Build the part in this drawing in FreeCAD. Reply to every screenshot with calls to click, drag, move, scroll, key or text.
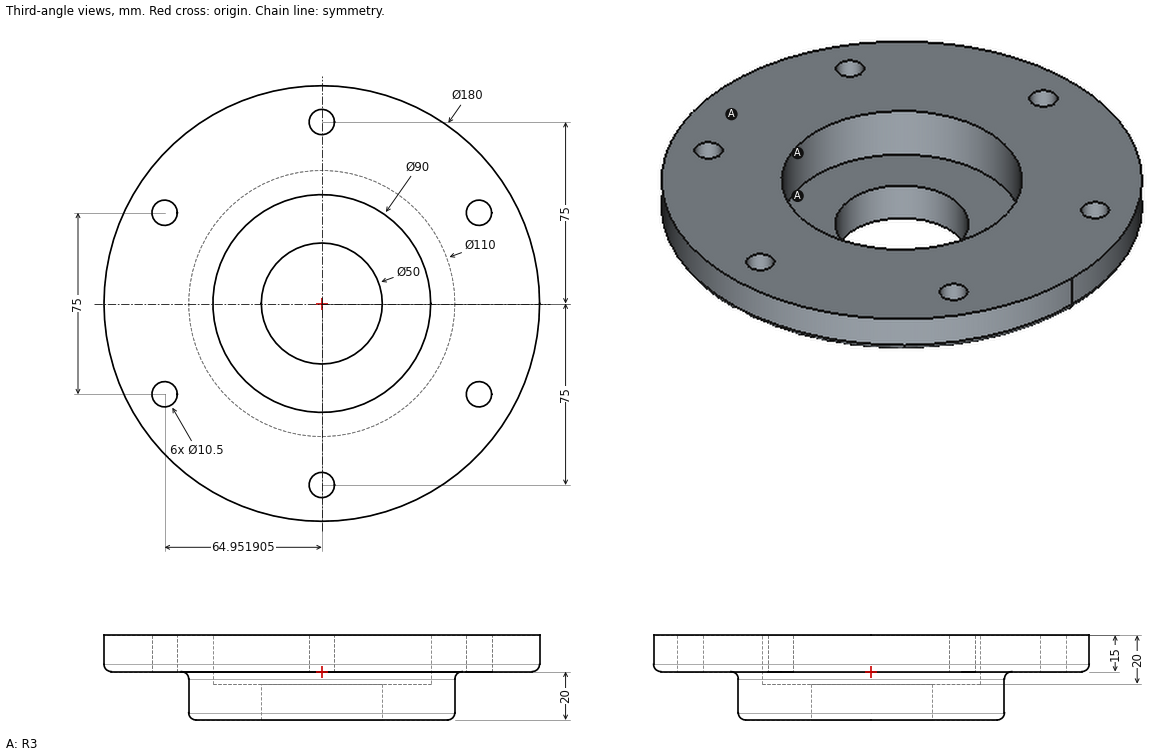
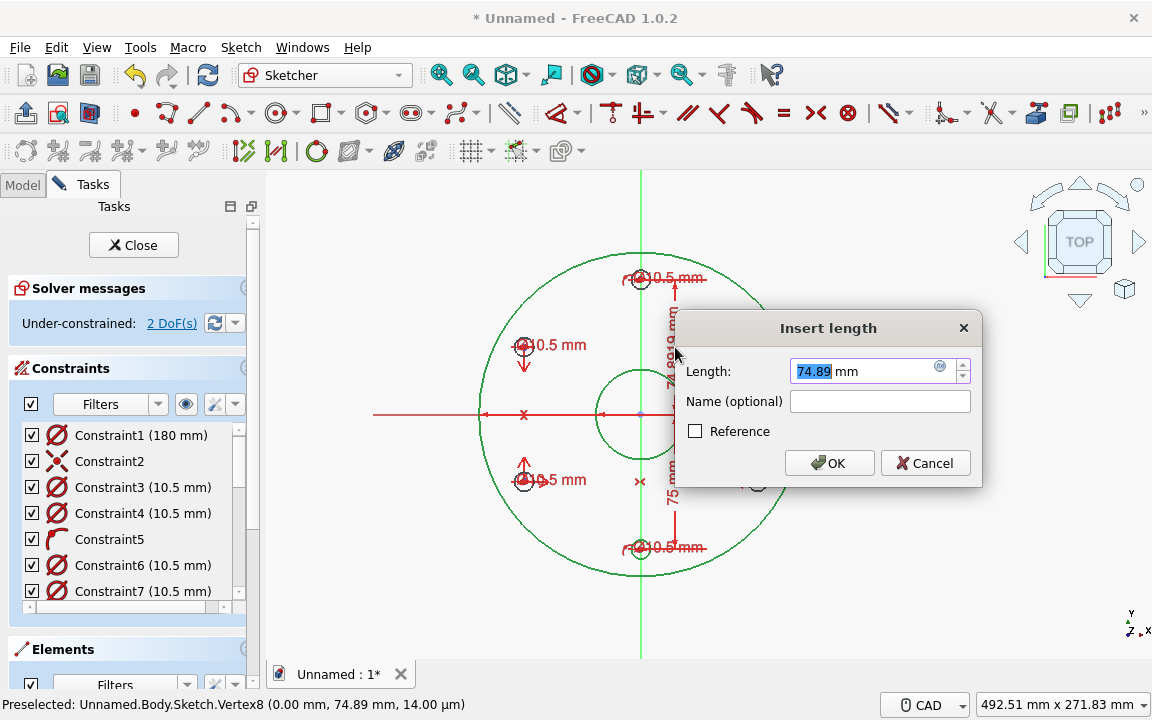
text(75)
key(Return)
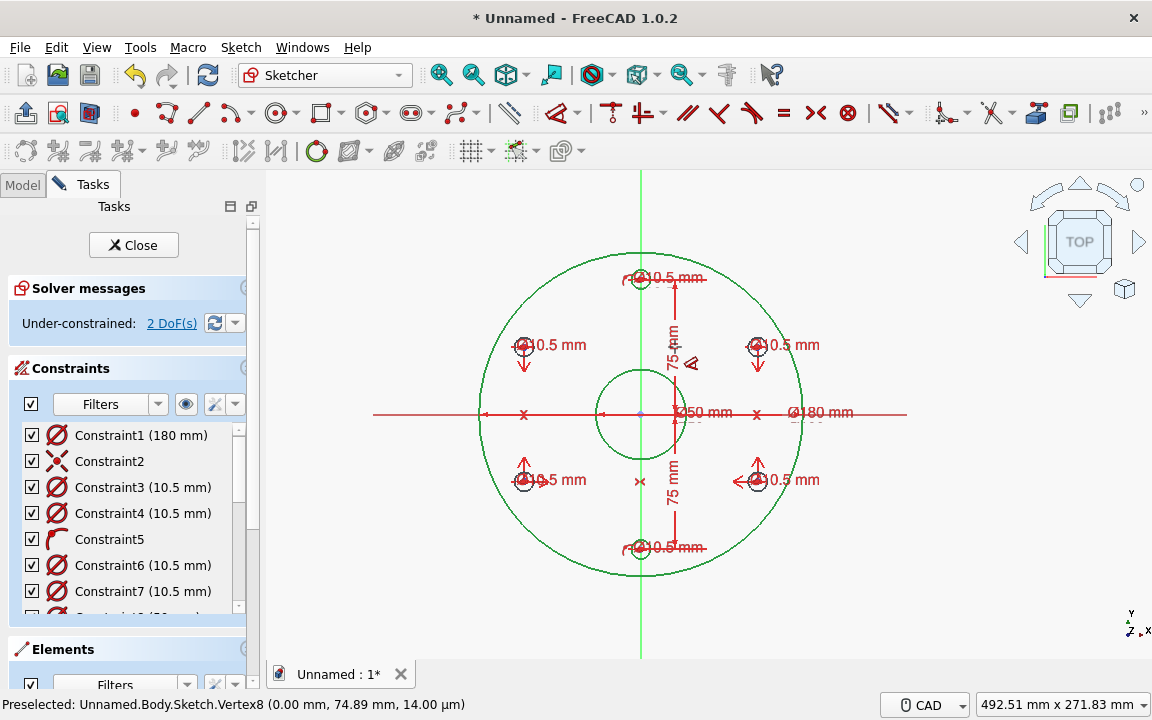
click(524, 482)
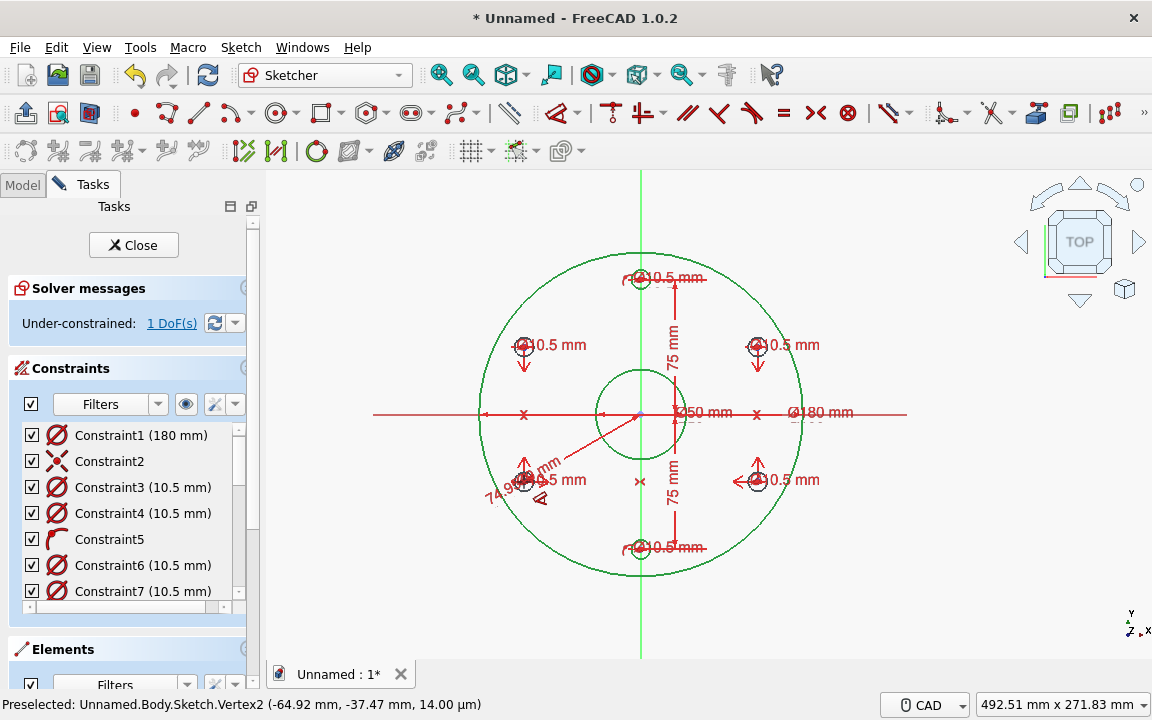
click(524, 347)
click(558, 383)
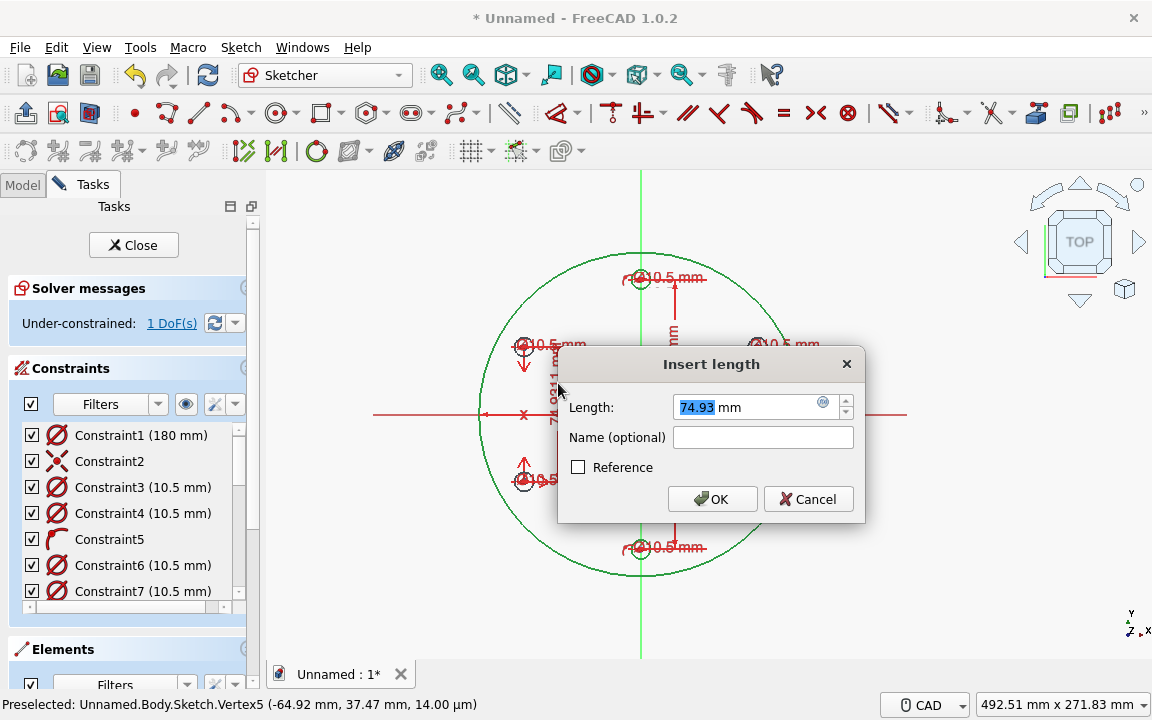
text(75)
key(Return)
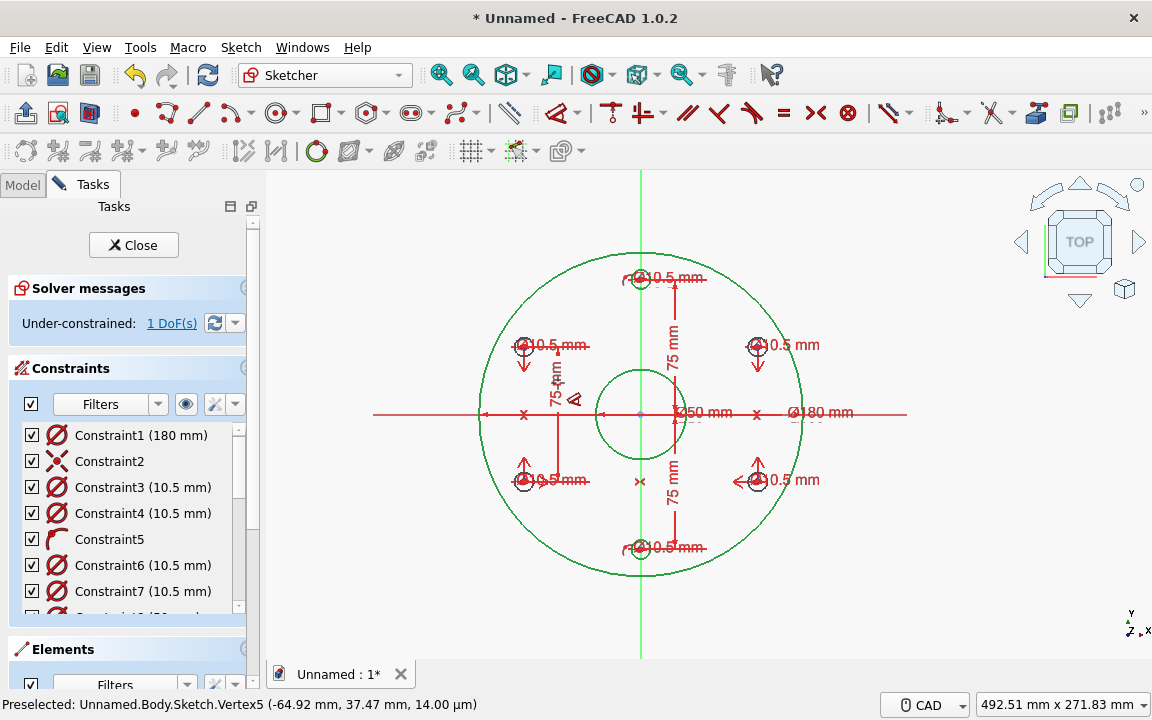
click(524, 482)
click(583, 516)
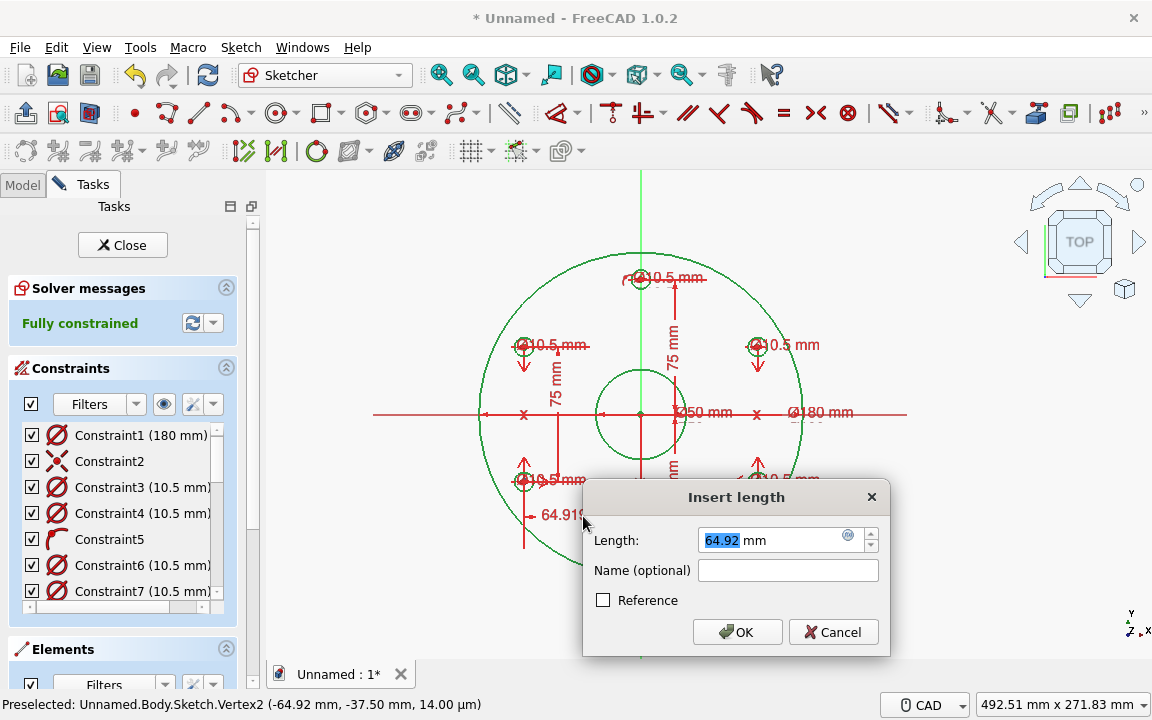
text(64.951905)
key(Return)
key(Escape)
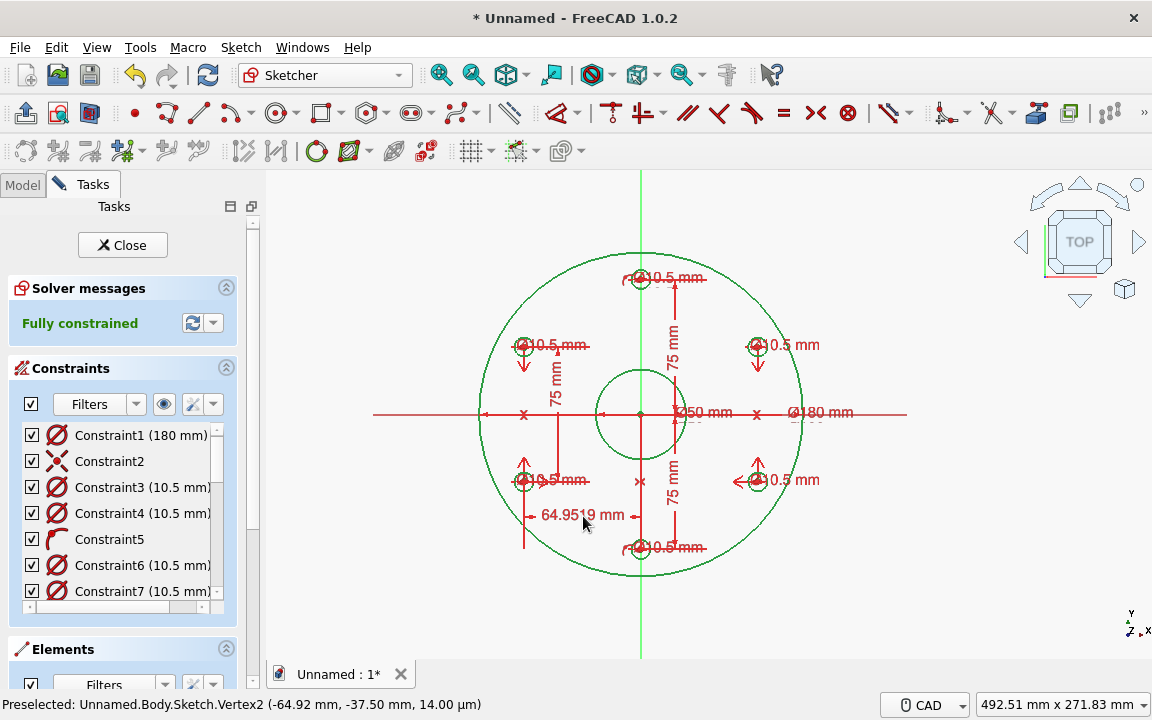
click(123, 245)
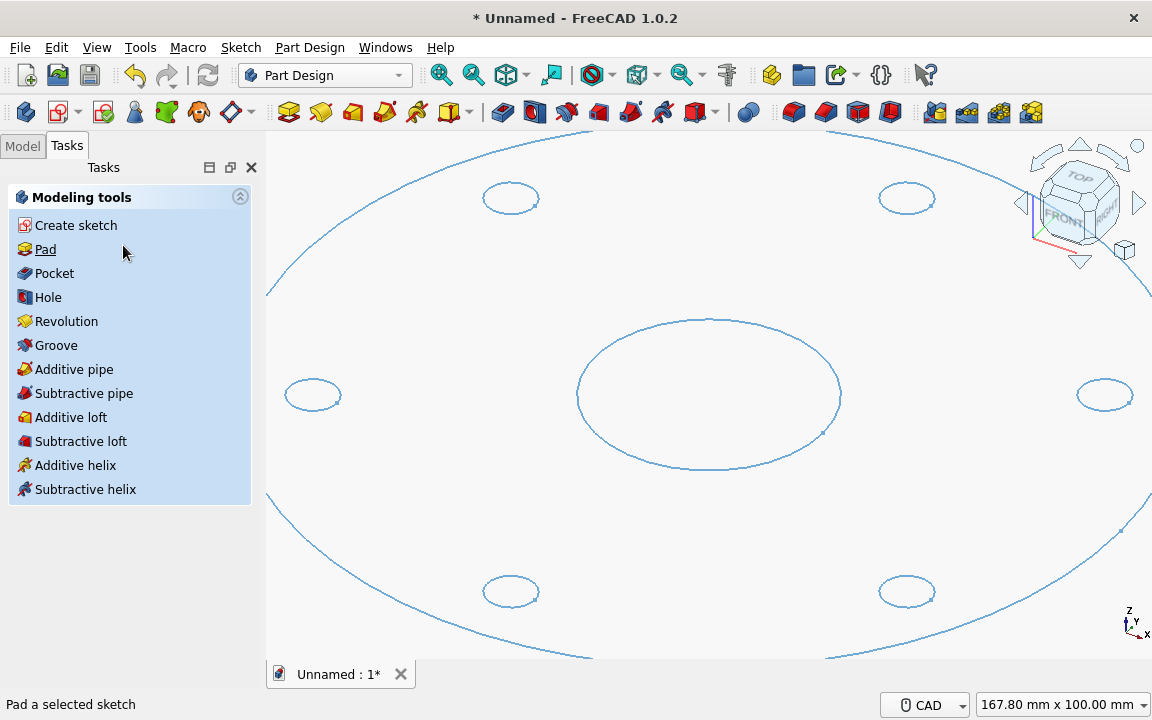
click(290, 112)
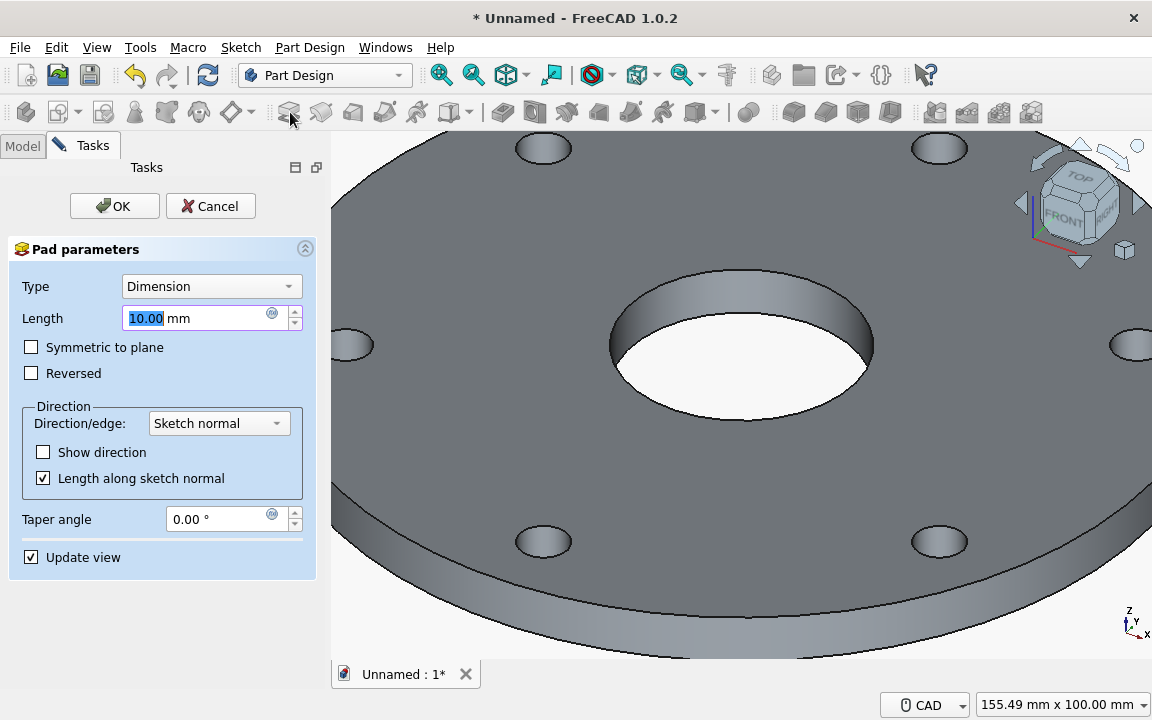
text(15)
key(Tab)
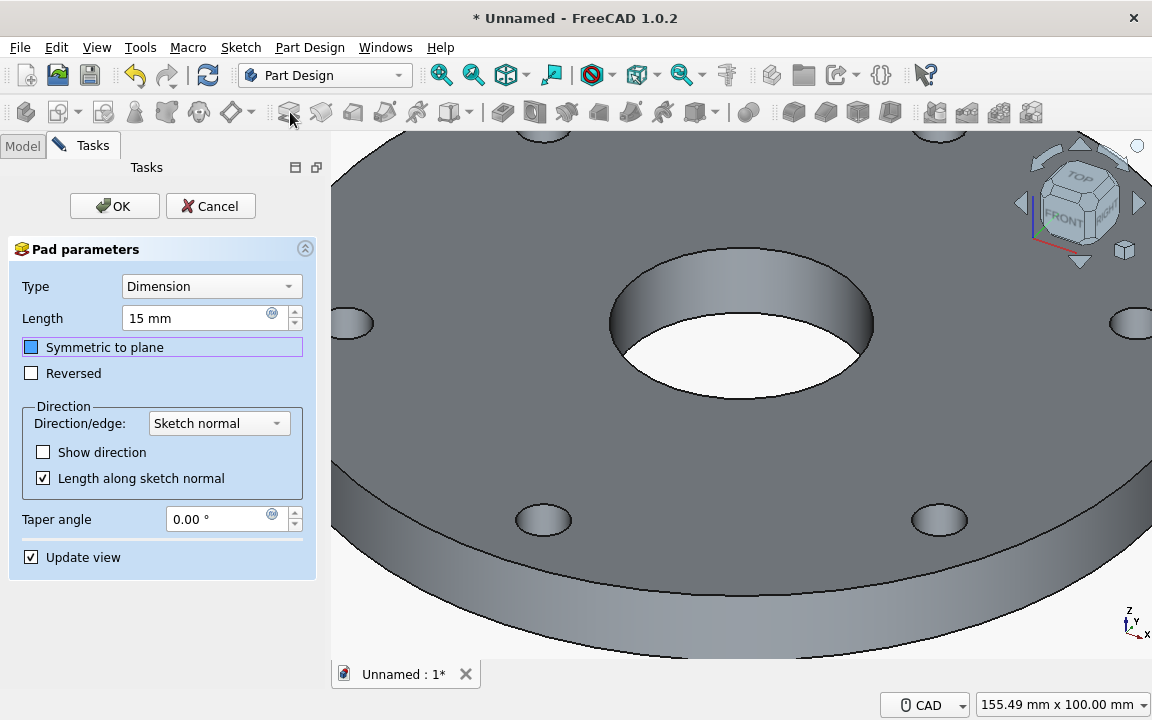
click(115, 206)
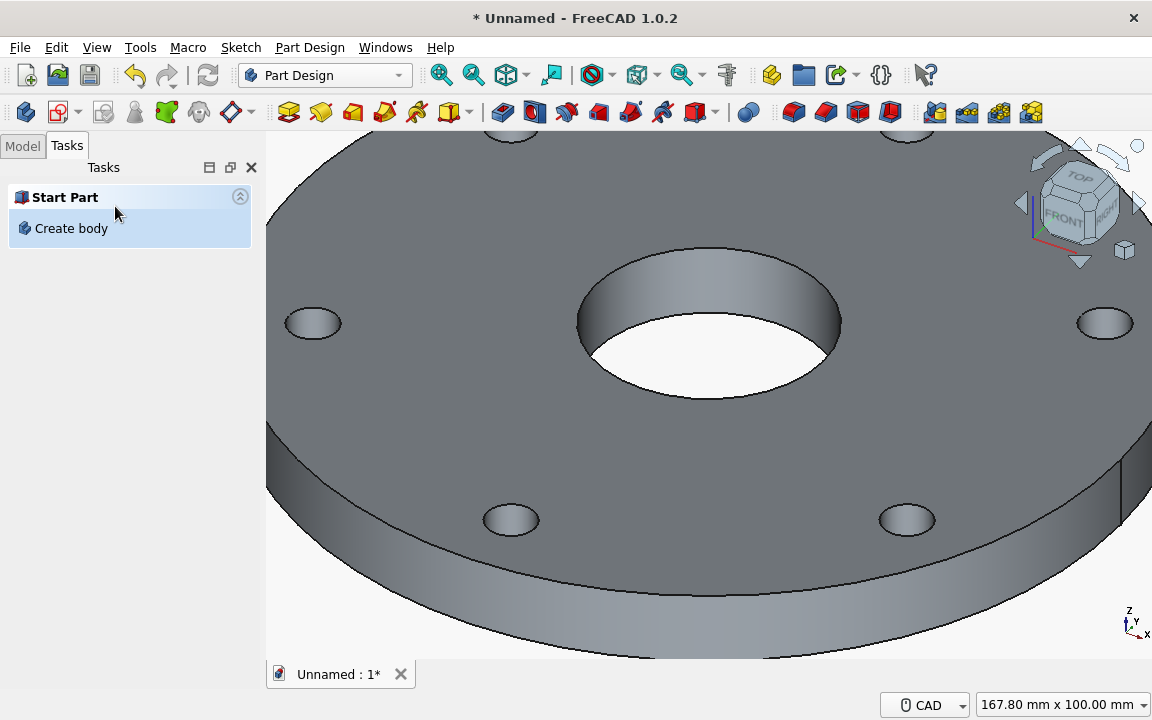
key(v)
key(f)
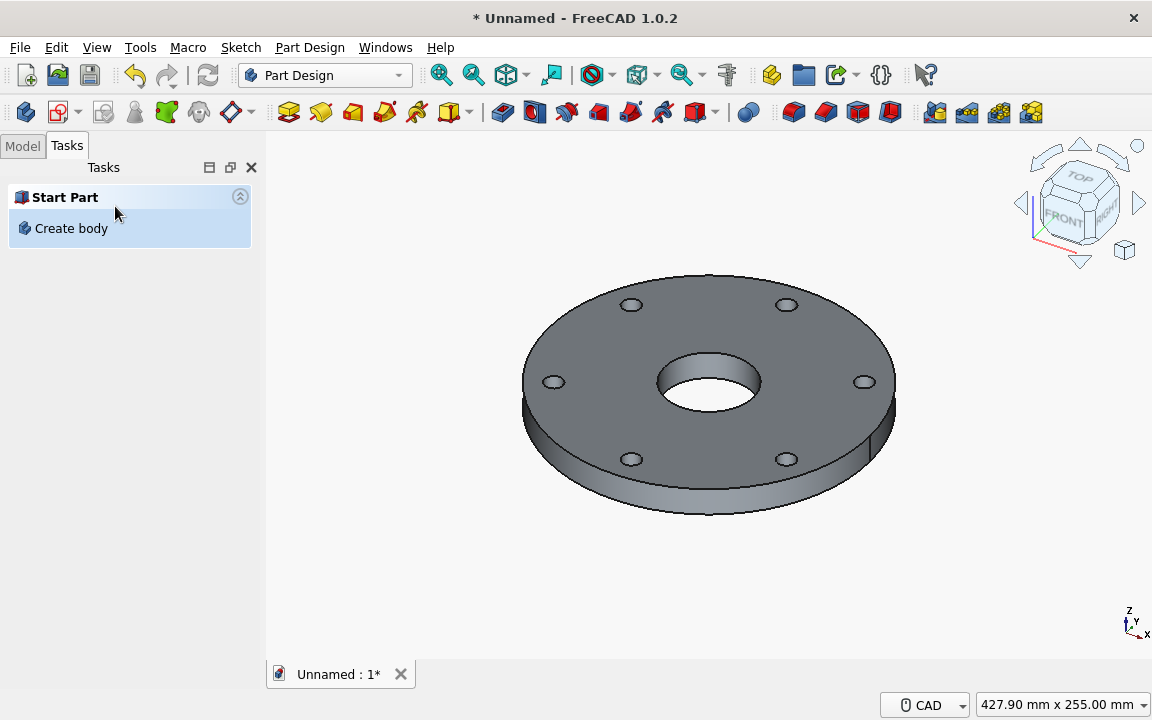
click(23, 145)